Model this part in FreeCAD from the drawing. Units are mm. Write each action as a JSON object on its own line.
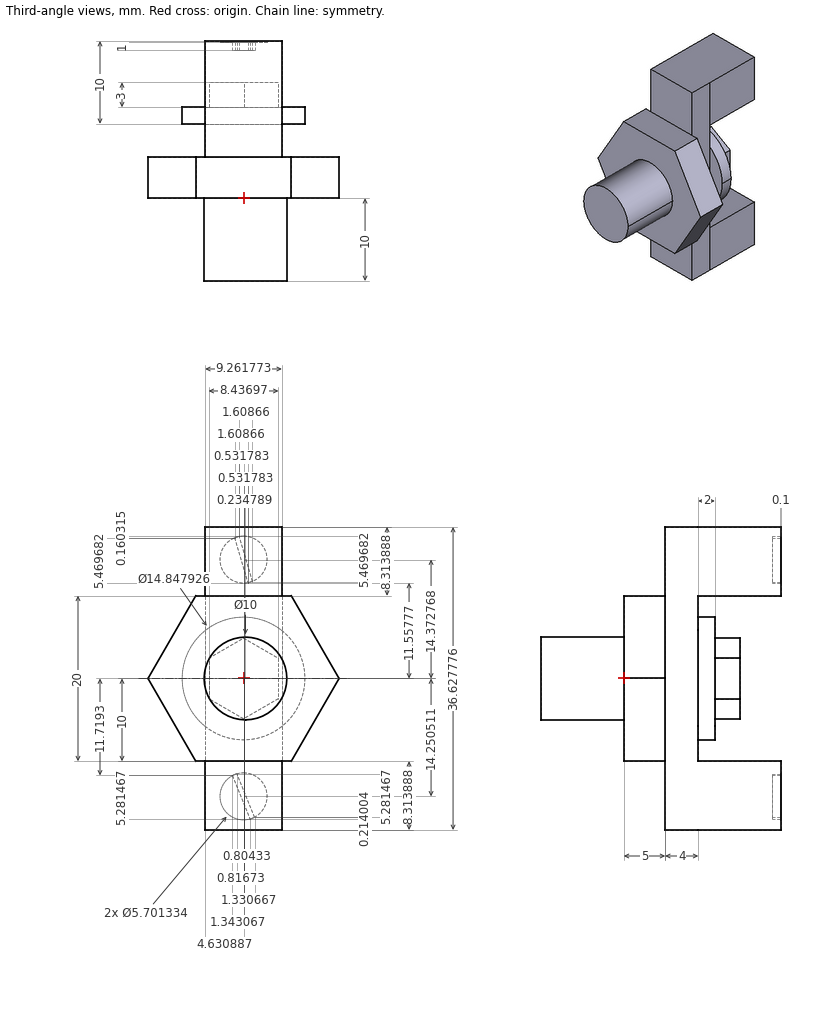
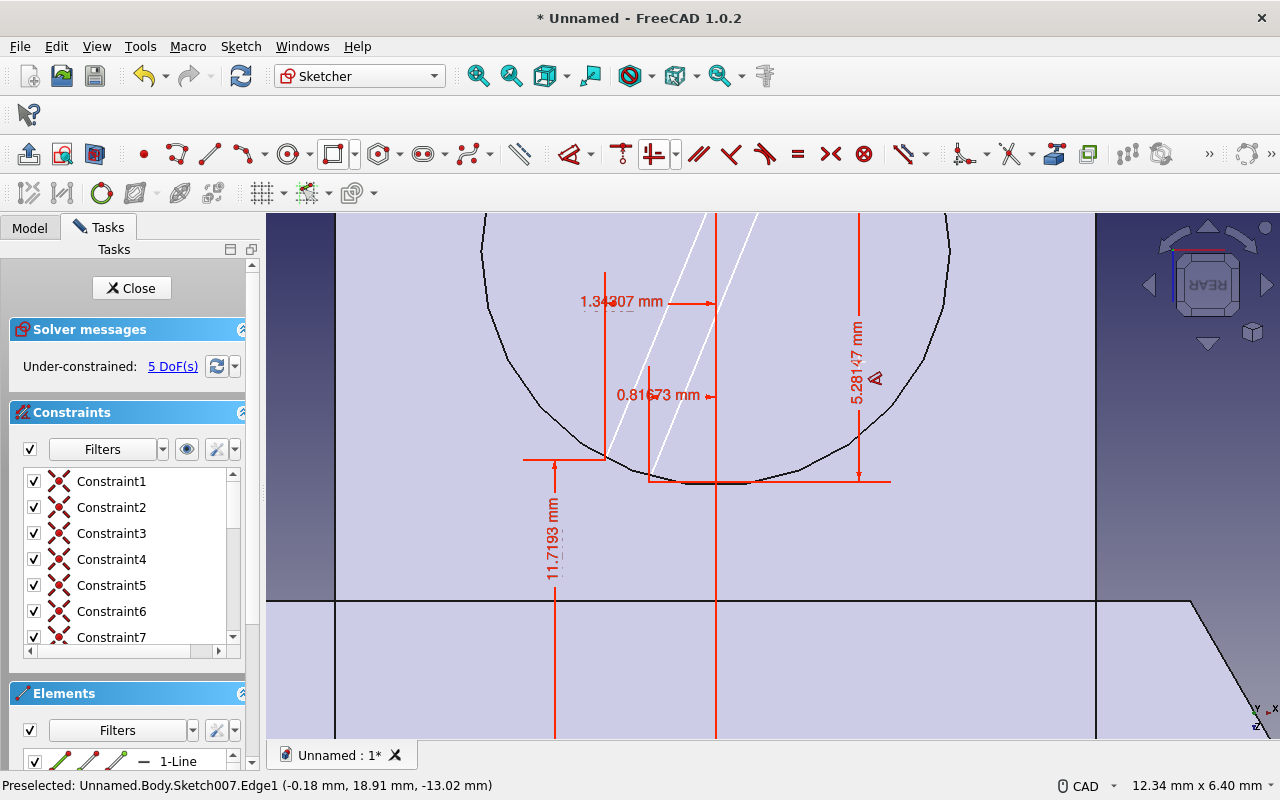
{"action": "scroll", "coordinate": [703, 357], "scroll_direction": "down", "scroll_amount": 11}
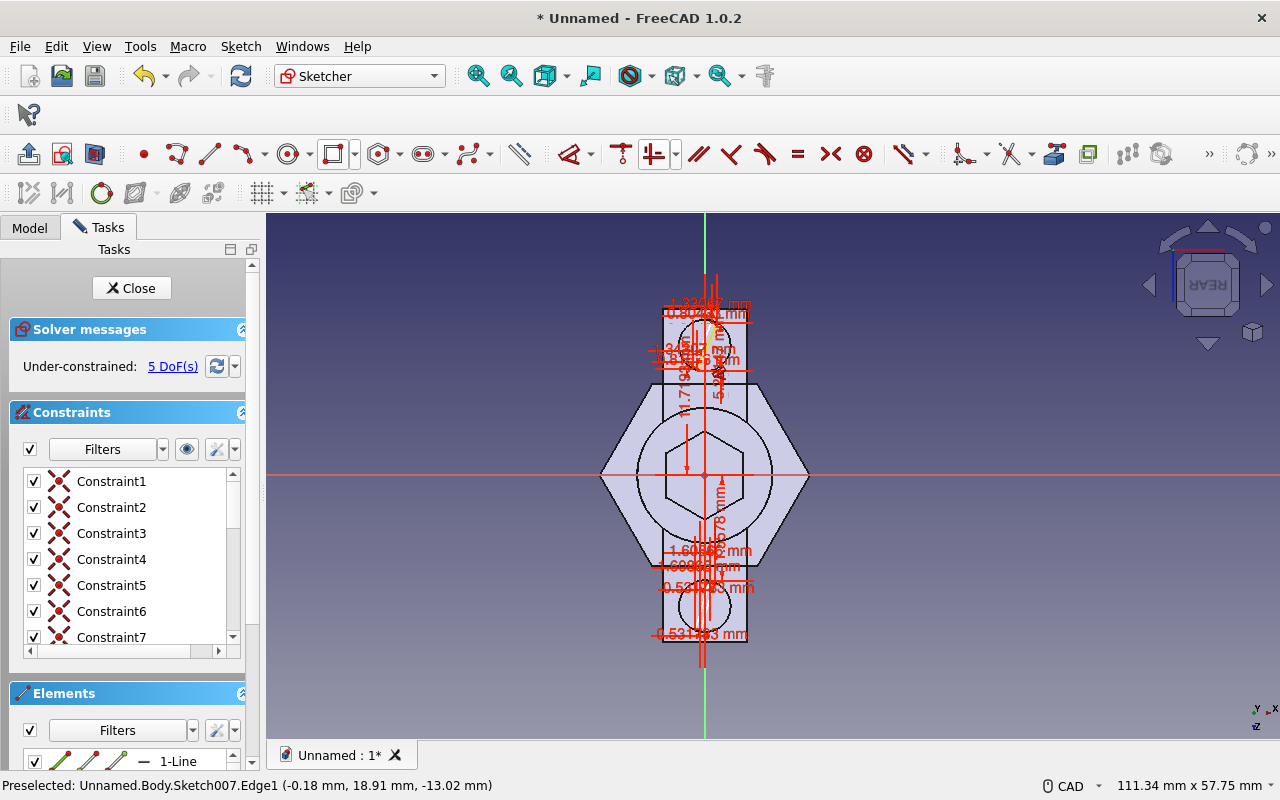
{"action": "scroll", "coordinate": [715, 322], "scroll_direction": "up", "scroll_amount": 16}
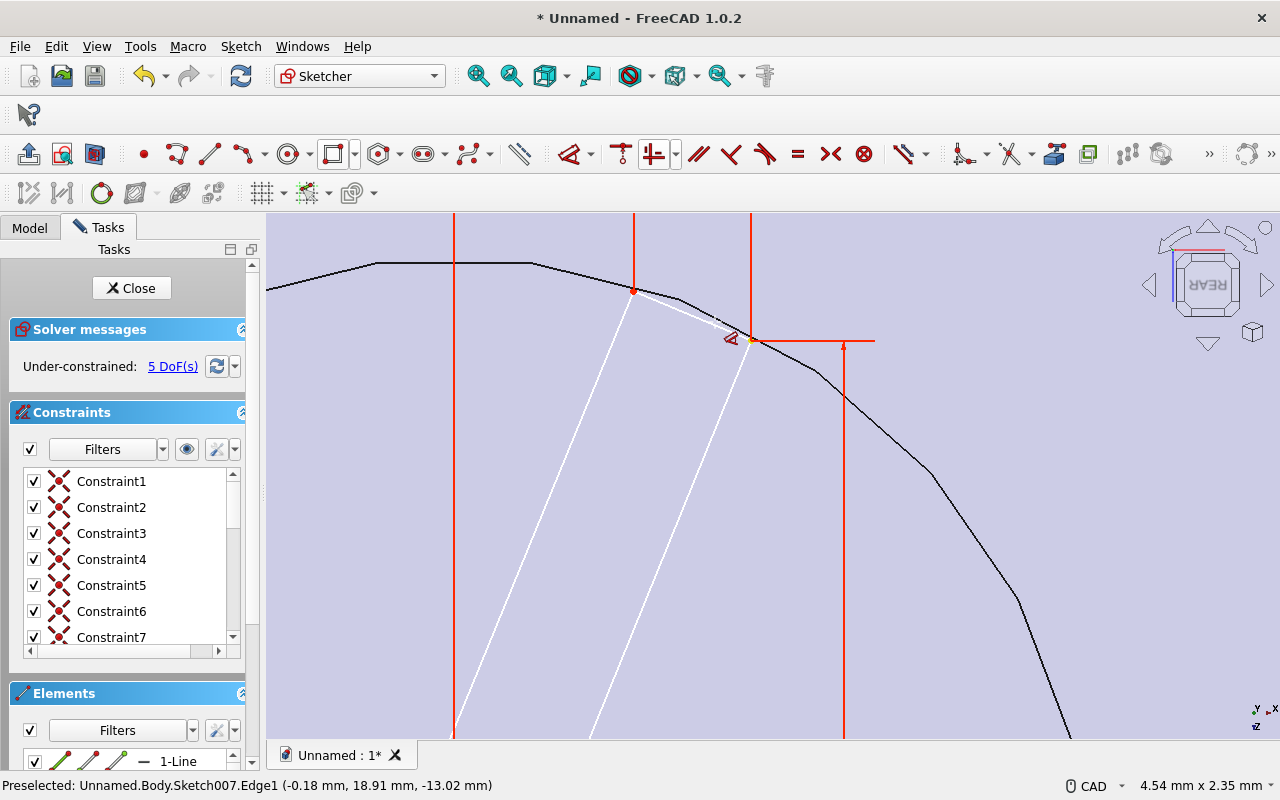
{"action": "left_click", "coordinate": [716, 326]}
{"action": "left_click", "coordinate": [785, 316]}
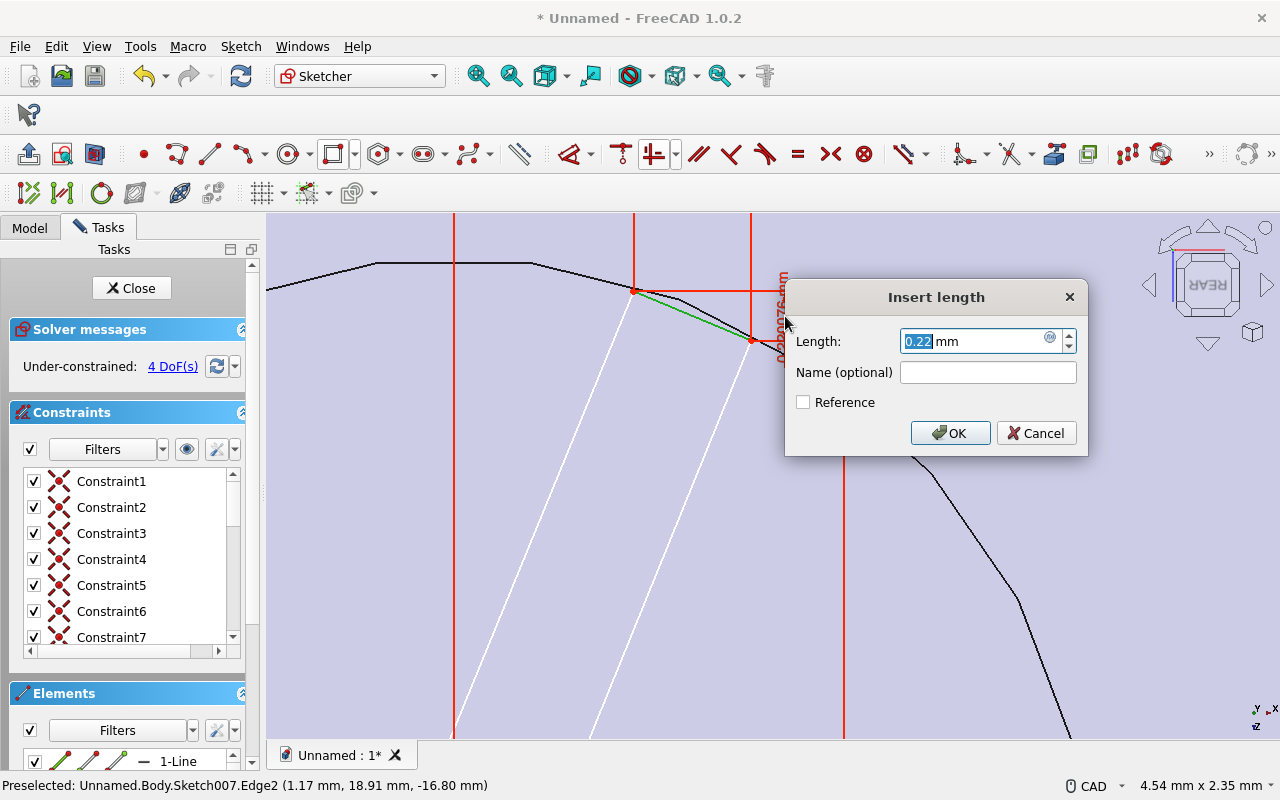
{"action": "type", "text": "0.214004"}
{"action": "key", "text": "Return"}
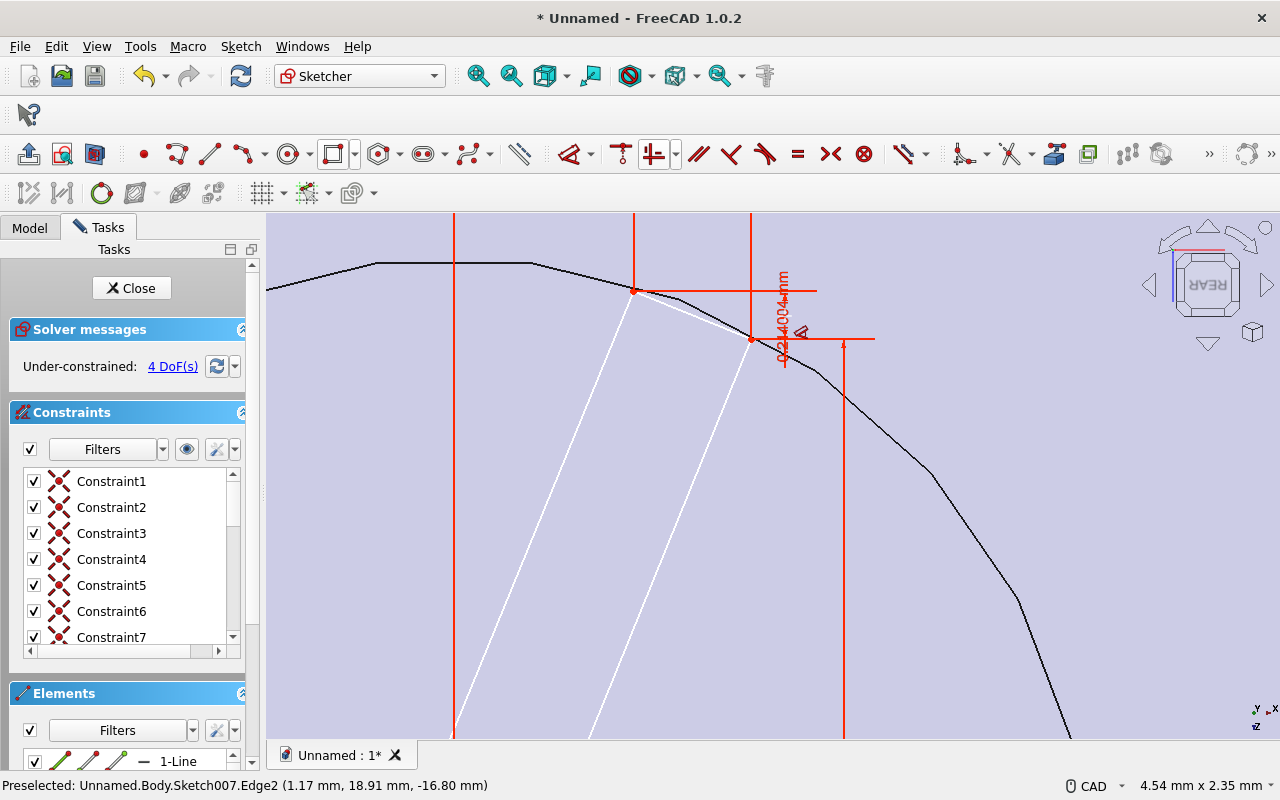
{"action": "left_click", "coordinate": [490, 642]}
{"action": "left_click", "coordinate": [668, 501]}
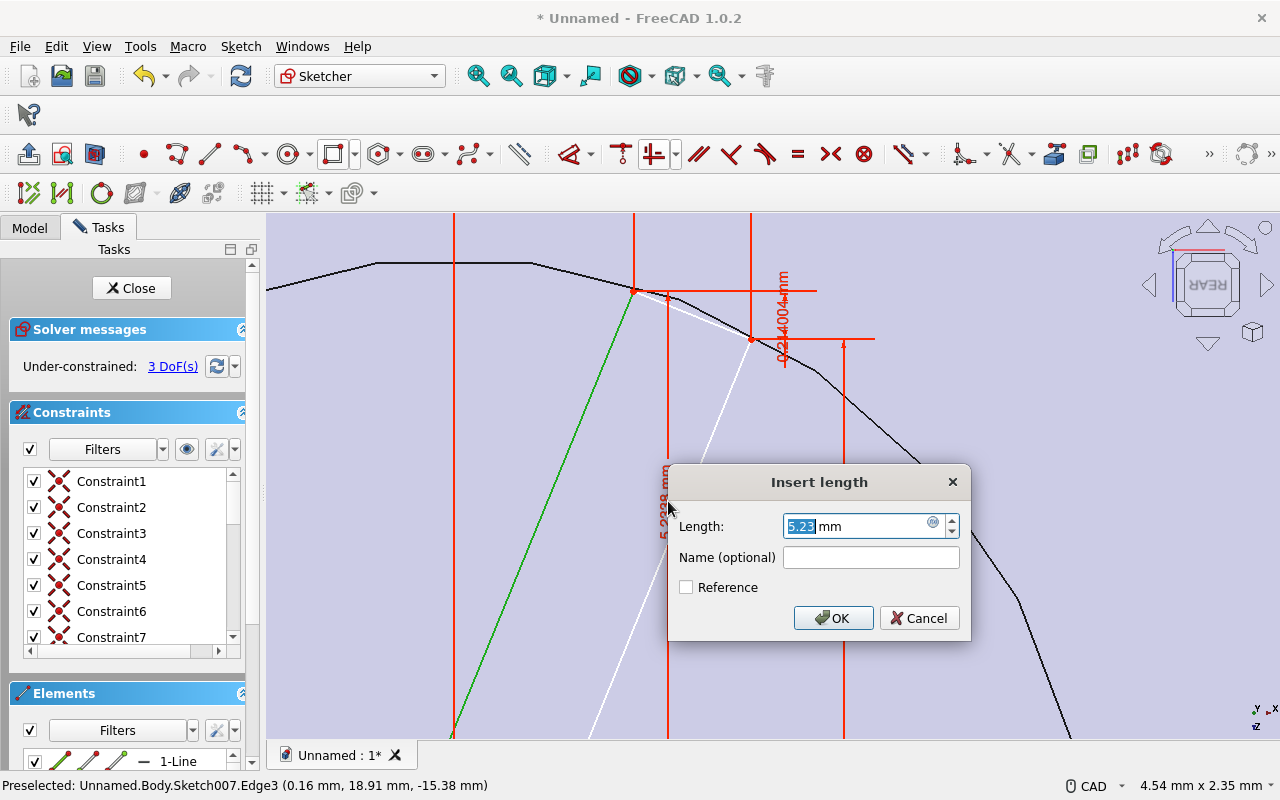
{"action": "type", "text": "5.281467"}
{"action": "key", "text": "Return"}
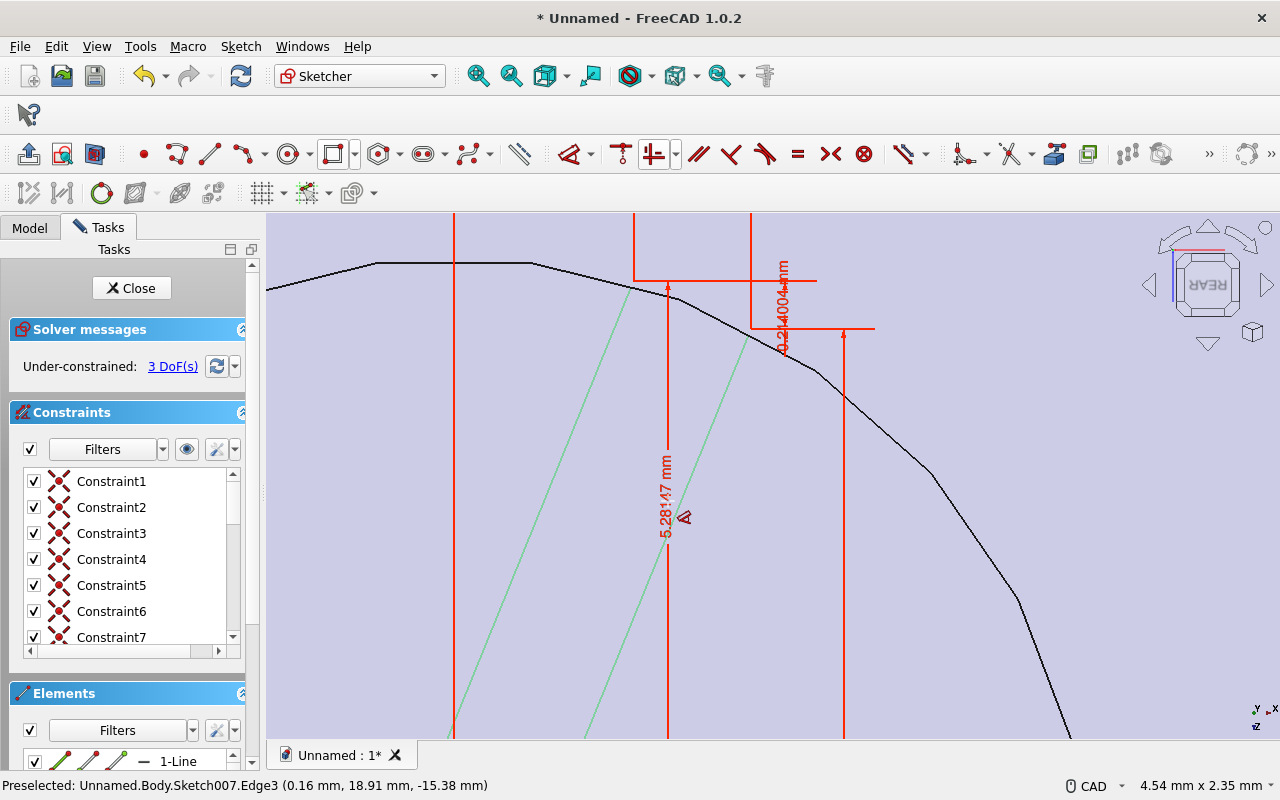
{"action": "scroll", "coordinate": [718, 286], "scroll_direction": "down", "scroll_amount": 15}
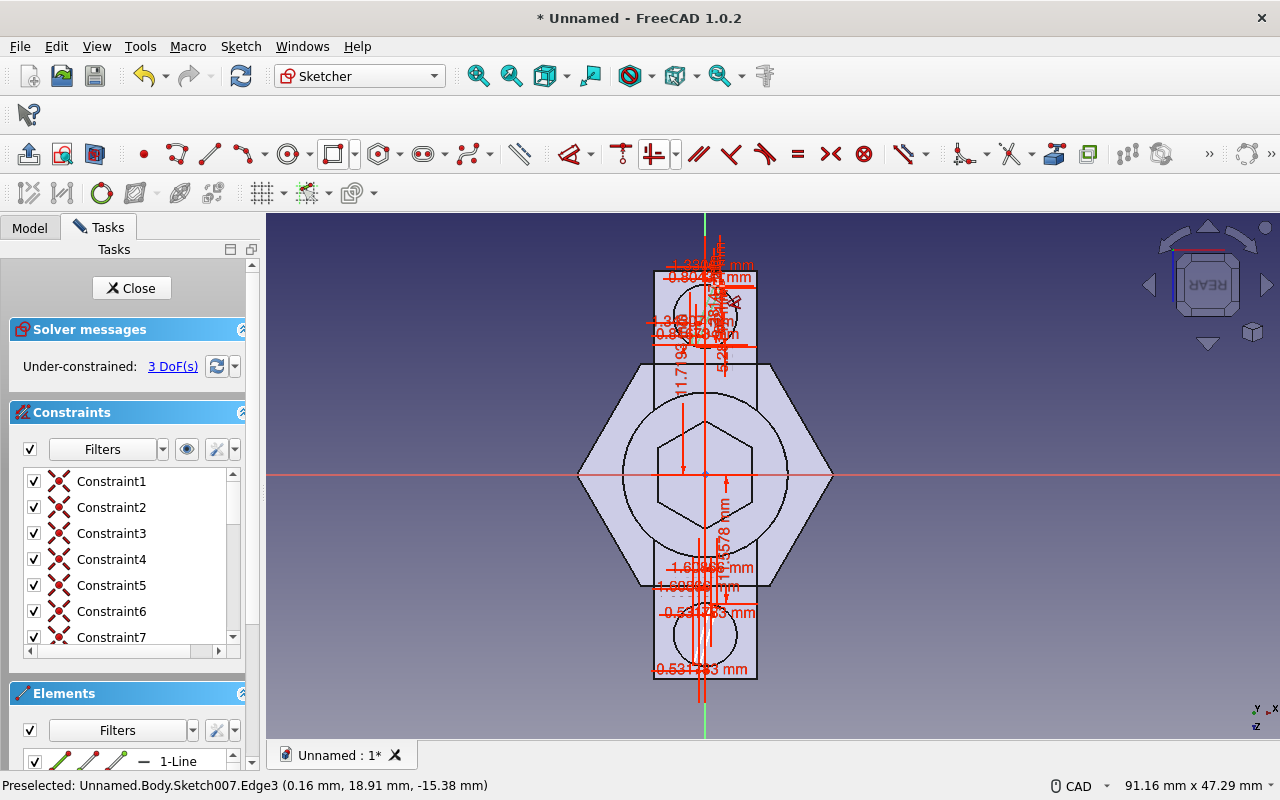
{"action": "scroll", "coordinate": [706, 622], "scroll_direction": "up", "scroll_amount": 14}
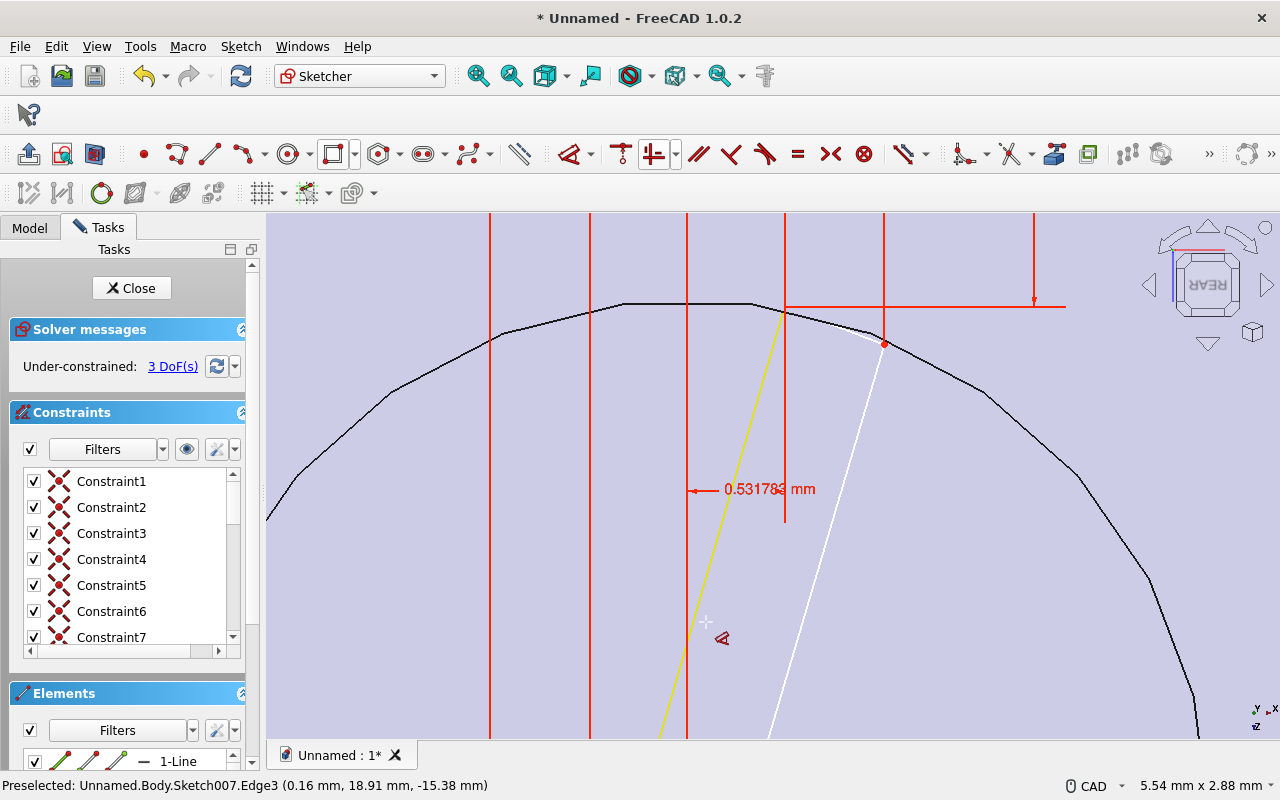
{"action": "left_click", "coordinate": [696, 611]}
{"action": "left_click", "coordinate": [456, 509]}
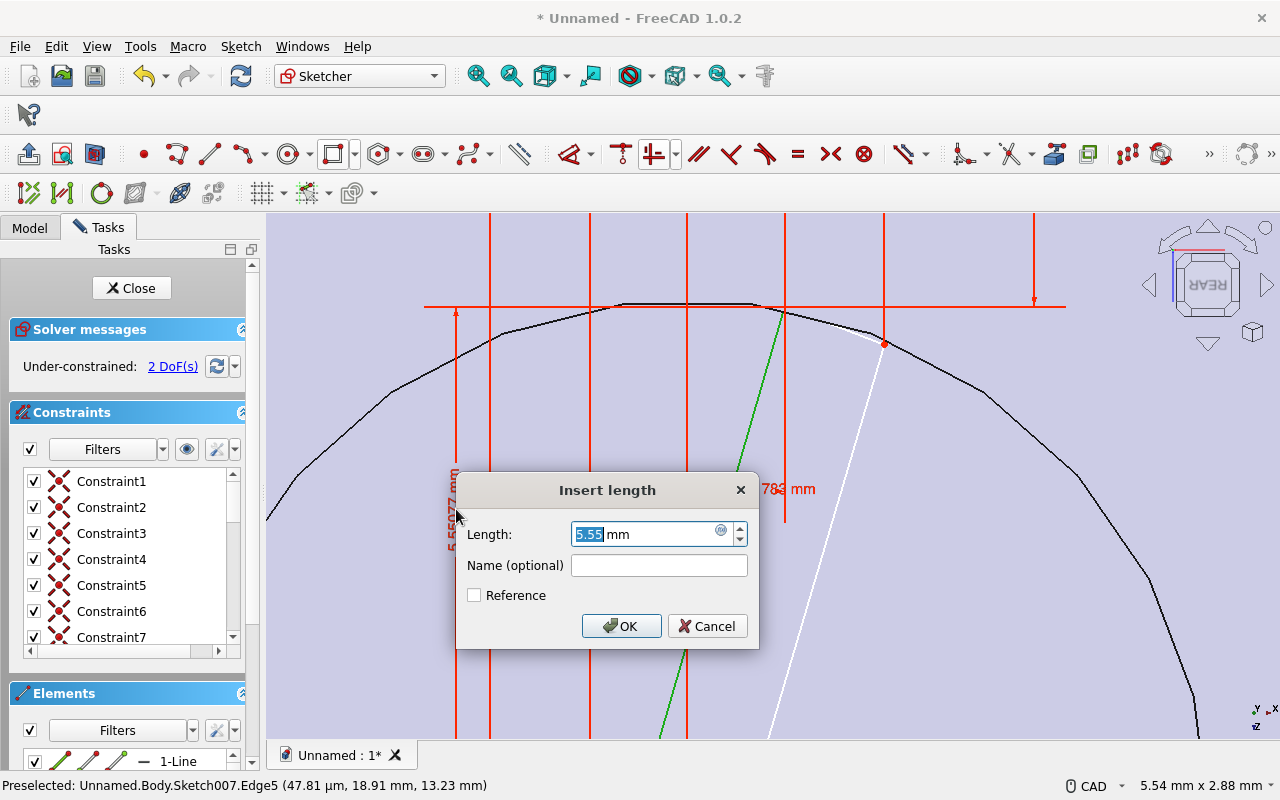
{"action": "type", "text": "5.469682"}
{"action": "key", "text": "Return"}